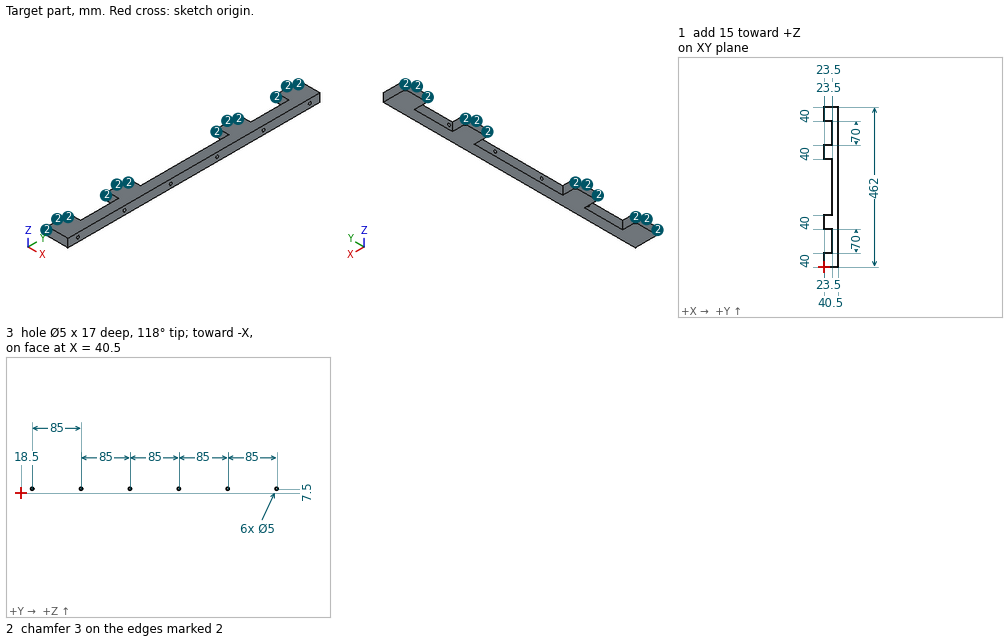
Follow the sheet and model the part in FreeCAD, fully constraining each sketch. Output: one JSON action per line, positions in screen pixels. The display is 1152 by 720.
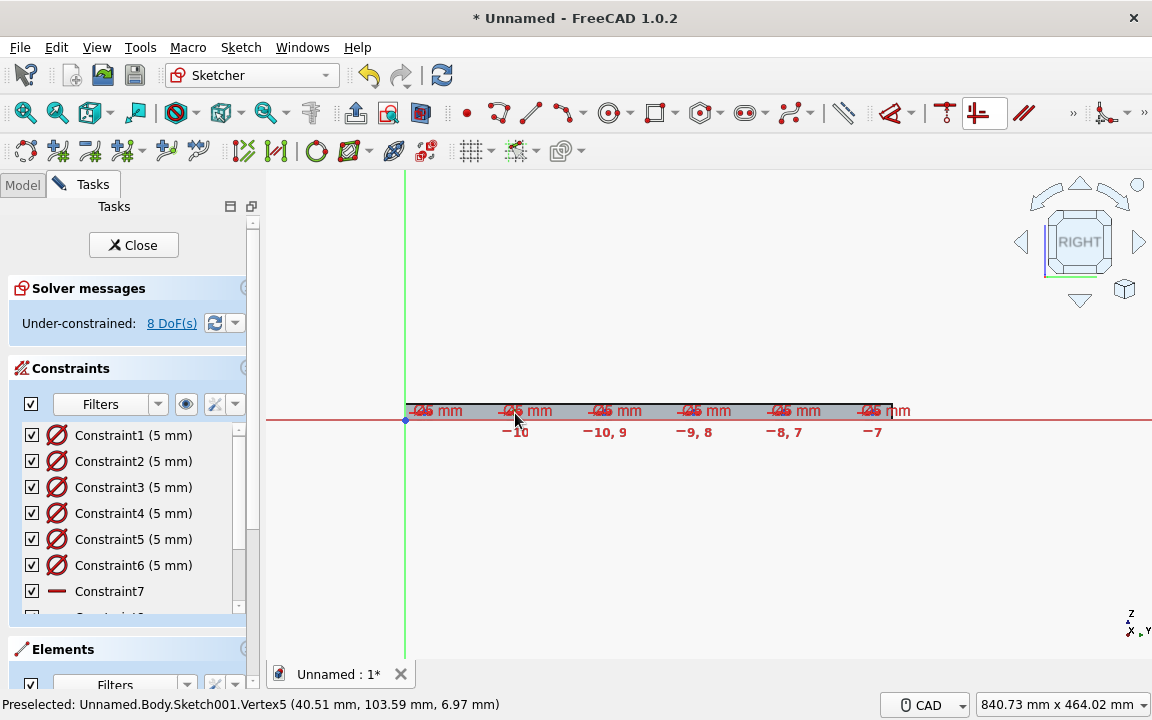
{"action": "left_click", "coordinate": [425, 413]}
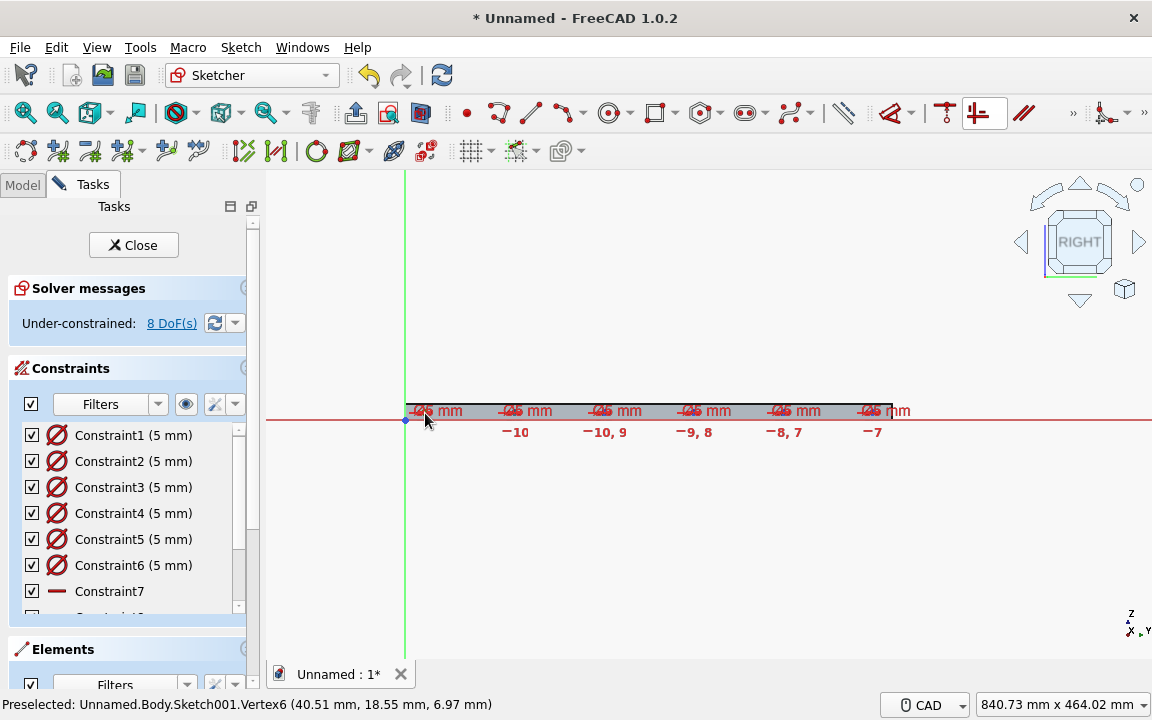
{"action": "key", "text": "h"}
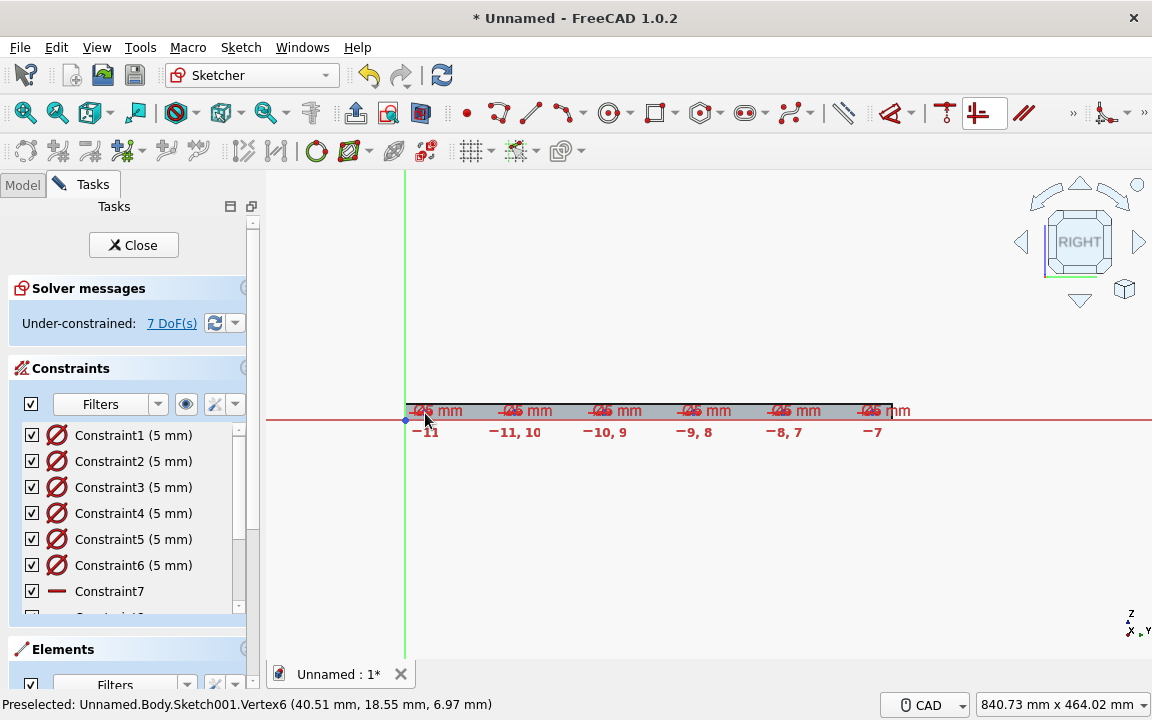
{"action": "left_click", "coordinate": [890, 114]}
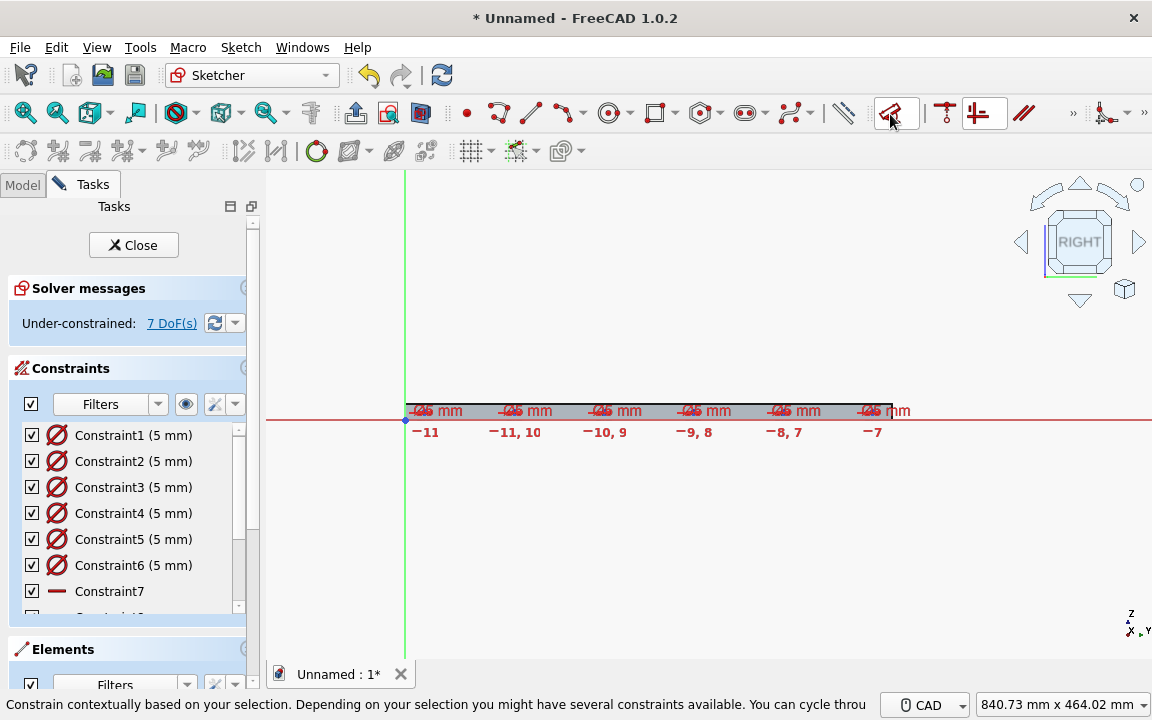
{"action": "scroll", "coordinate": [873, 413], "scroll_direction": "up", "scroll_amount": 9}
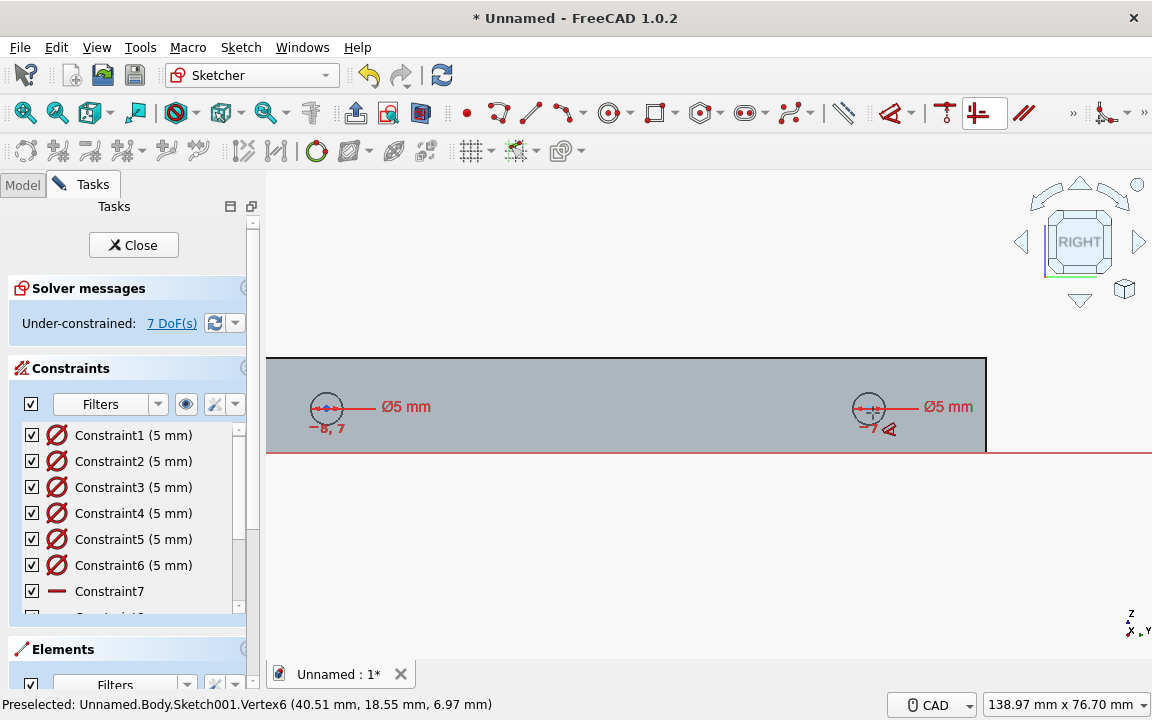
{"action": "left_click", "coordinate": [869, 409]}
{"action": "left_click", "coordinate": [903, 431]}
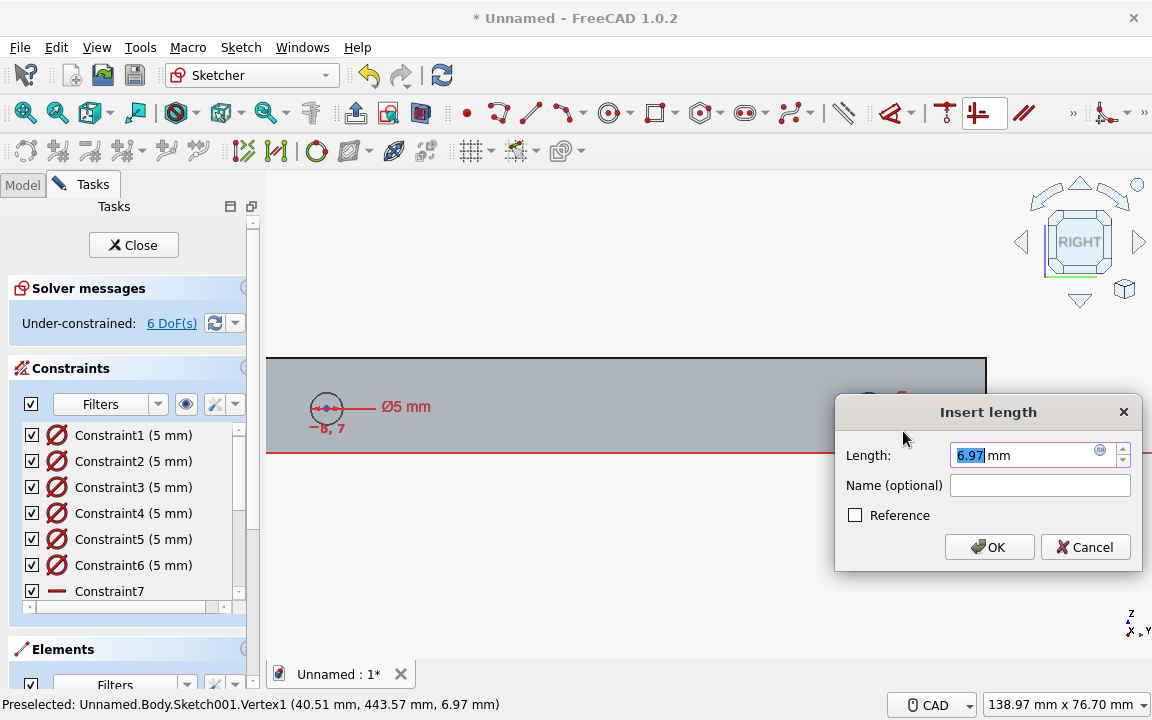
{"action": "type", "text": "7.5"}
{"action": "key", "text": "Return"}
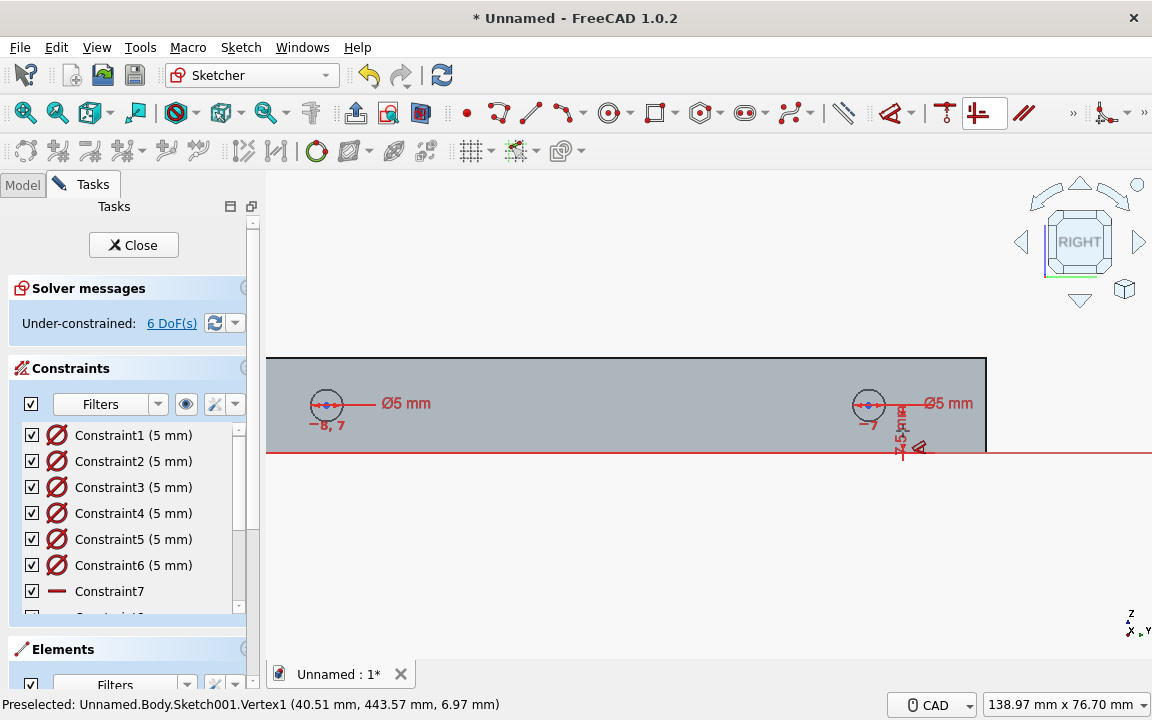
{"action": "scroll", "coordinate": [874, 413], "scroll_direction": "down", "scroll_amount": 9}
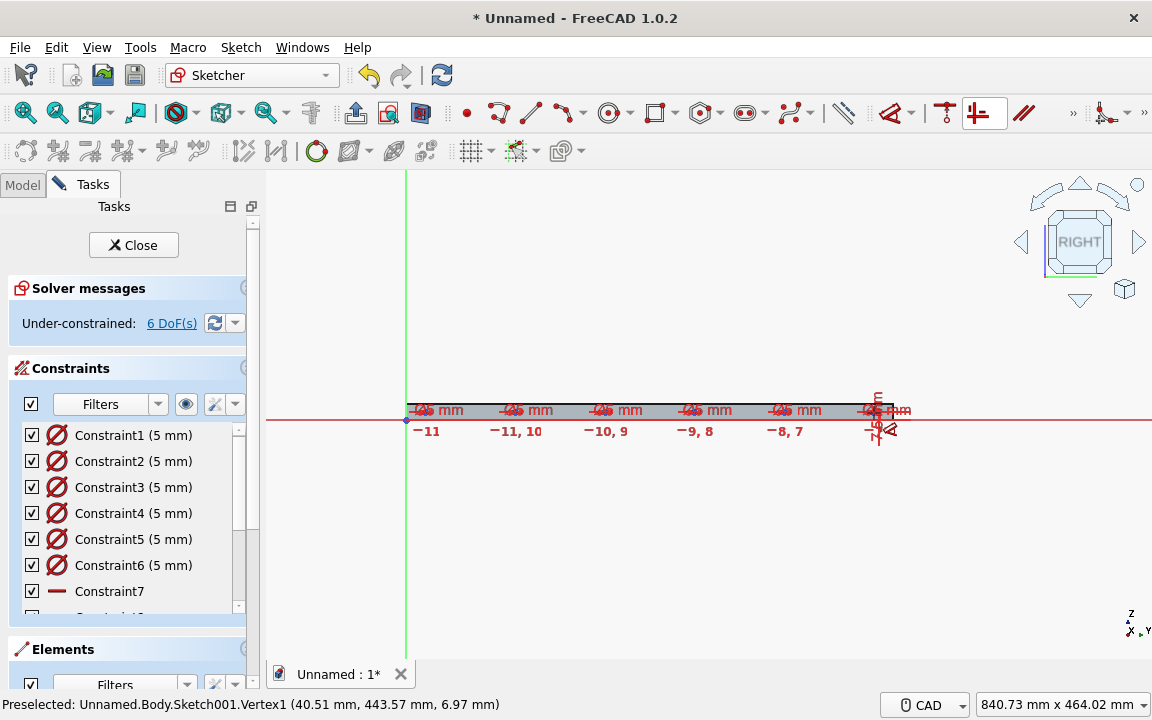
{"action": "left_click", "coordinate": [874, 412]}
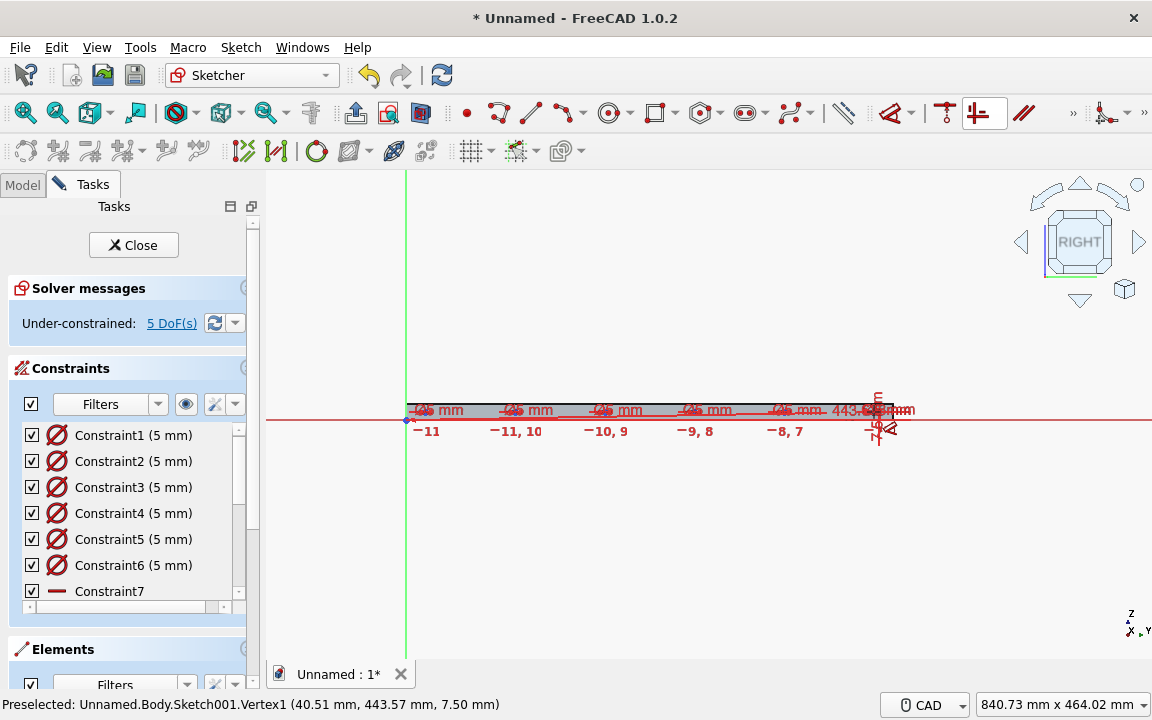
{"action": "left_click", "coordinate": [784, 412]}
{"action": "left_click", "coordinate": [829, 378]}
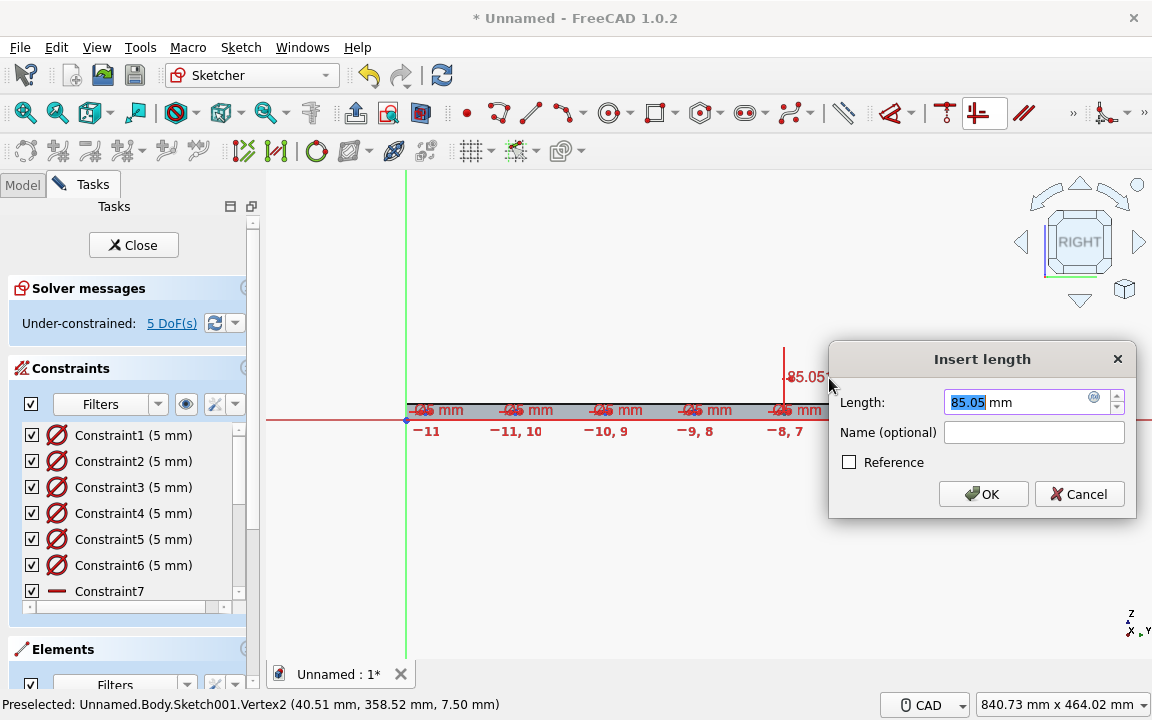
{"action": "type", "text": "85"}
{"action": "key", "text": "Return"}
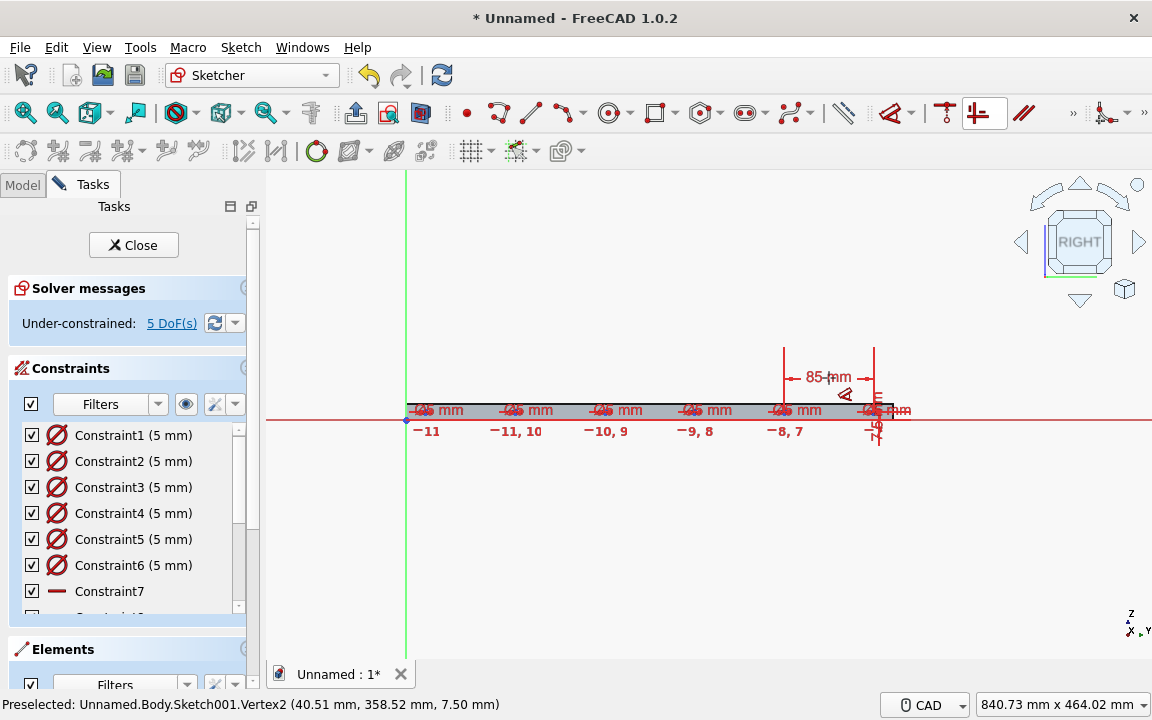
{"action": "left_click", "coordinate": [784, 412]}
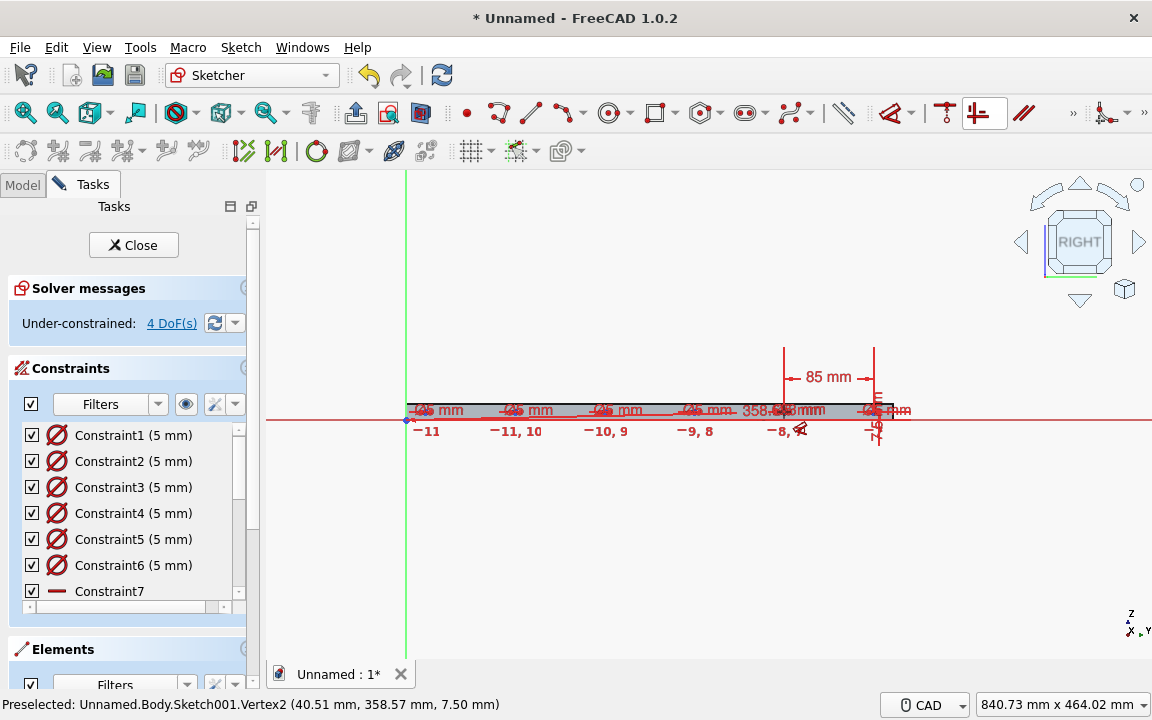
{"action": "left_click", "coordinate": [694, 412]}
{"action": "left_click", "coordinate": [739, 378]}